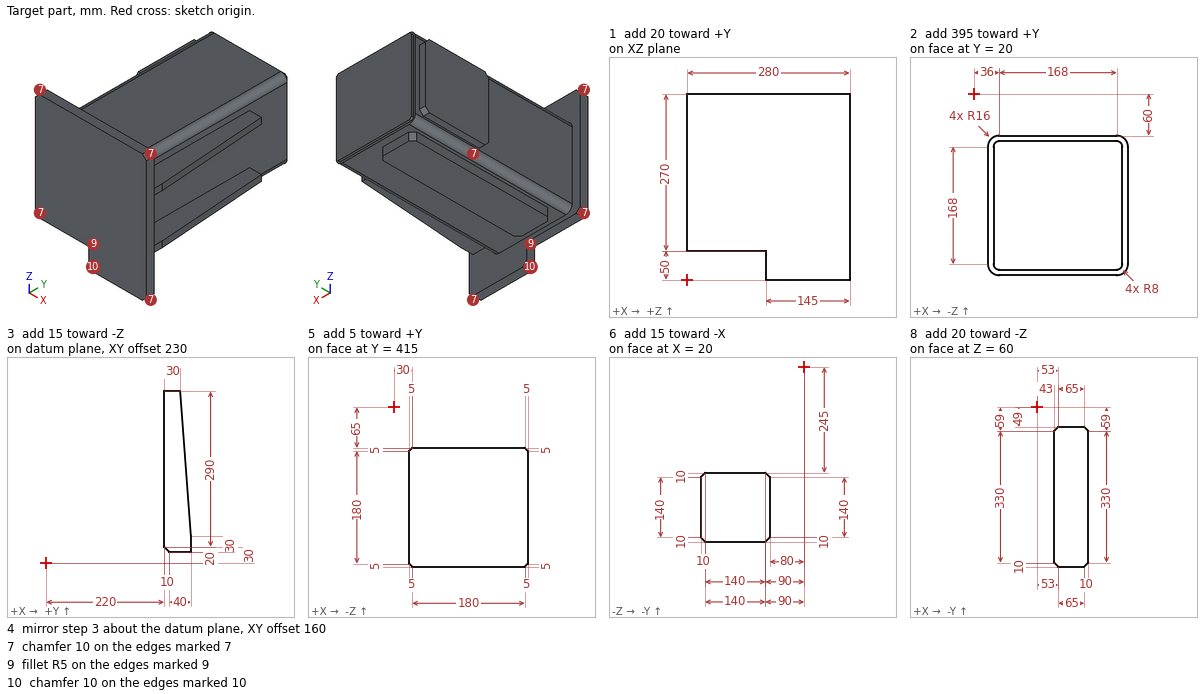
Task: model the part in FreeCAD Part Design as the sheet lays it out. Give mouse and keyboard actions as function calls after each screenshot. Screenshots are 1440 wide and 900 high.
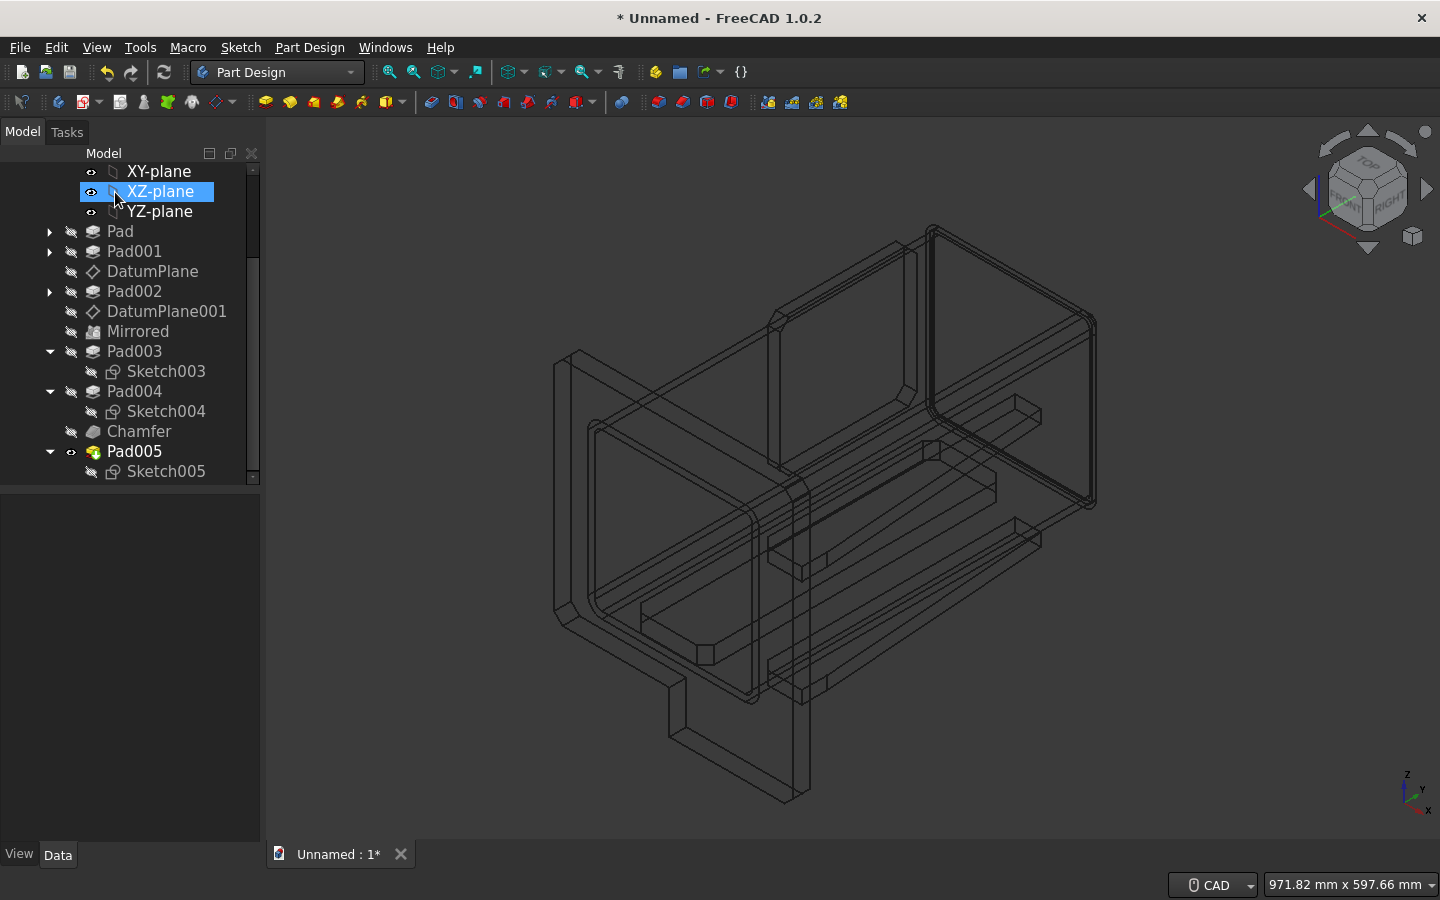
click(678, 682)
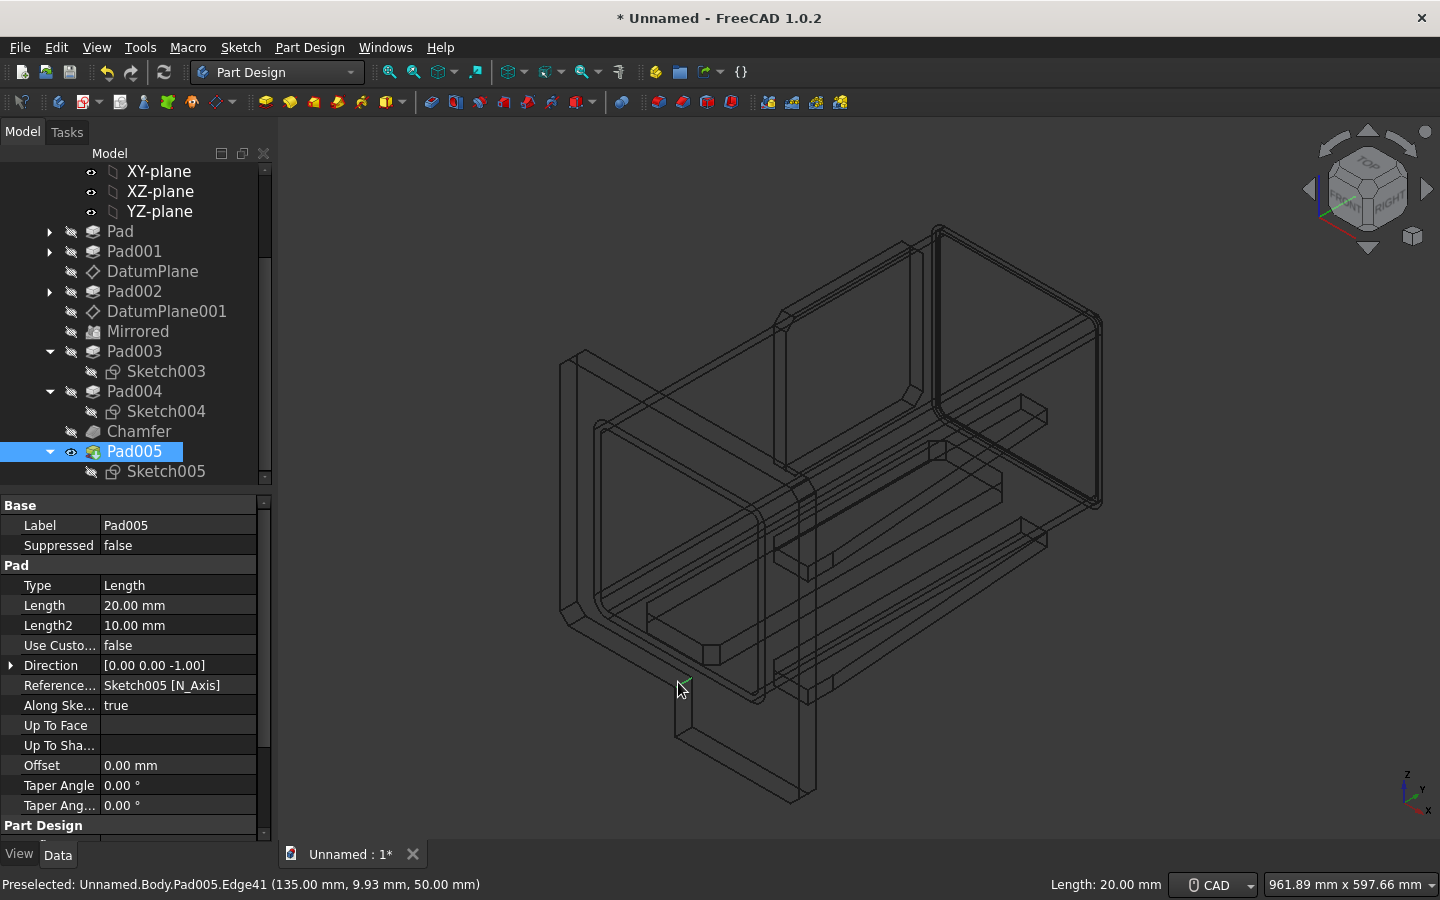
key(v)
key(1)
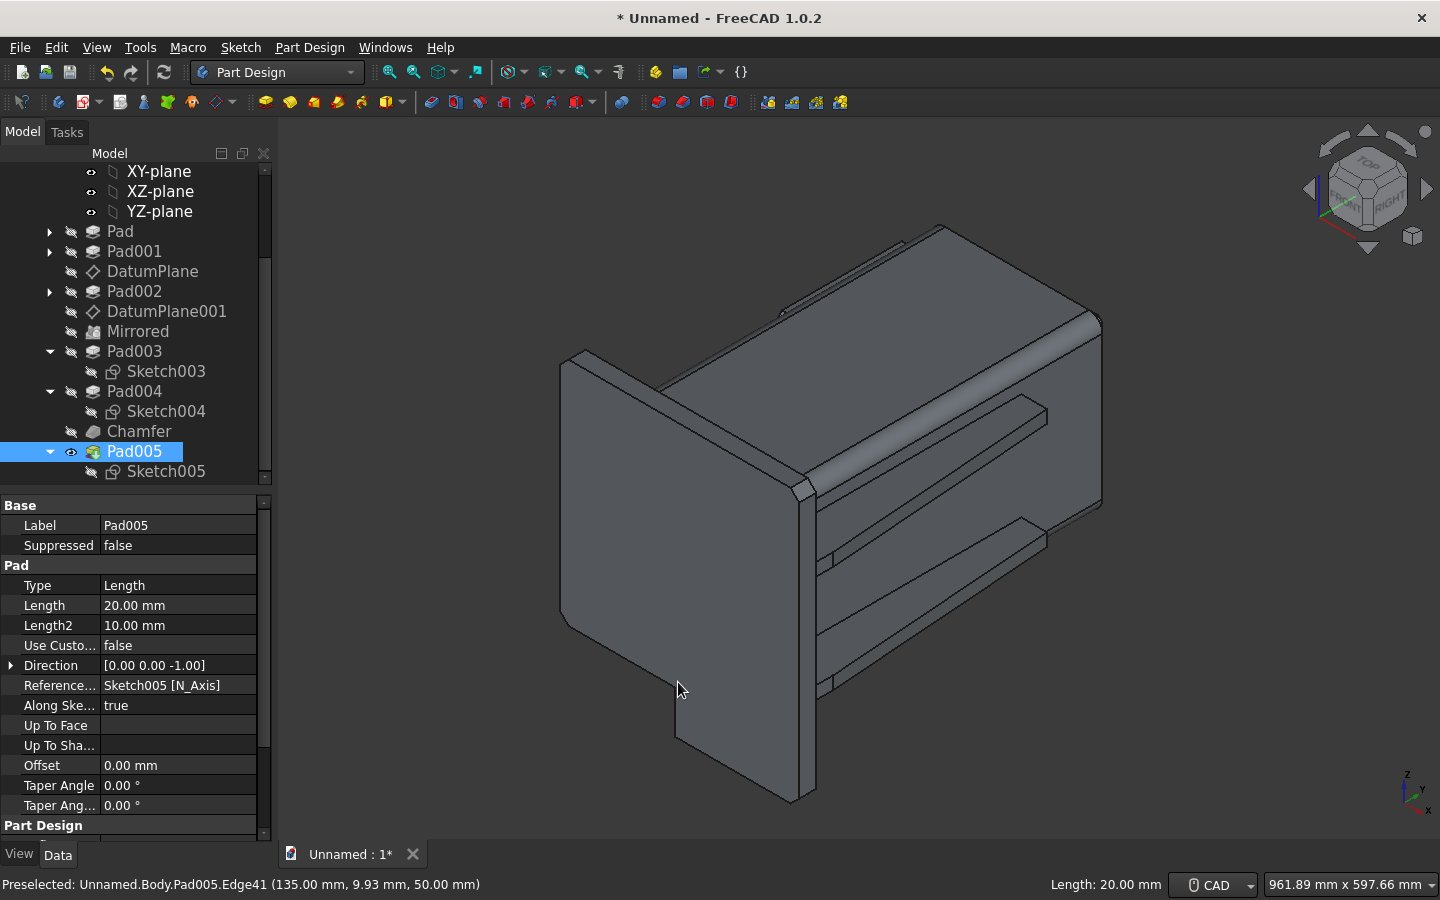
click(660, 102)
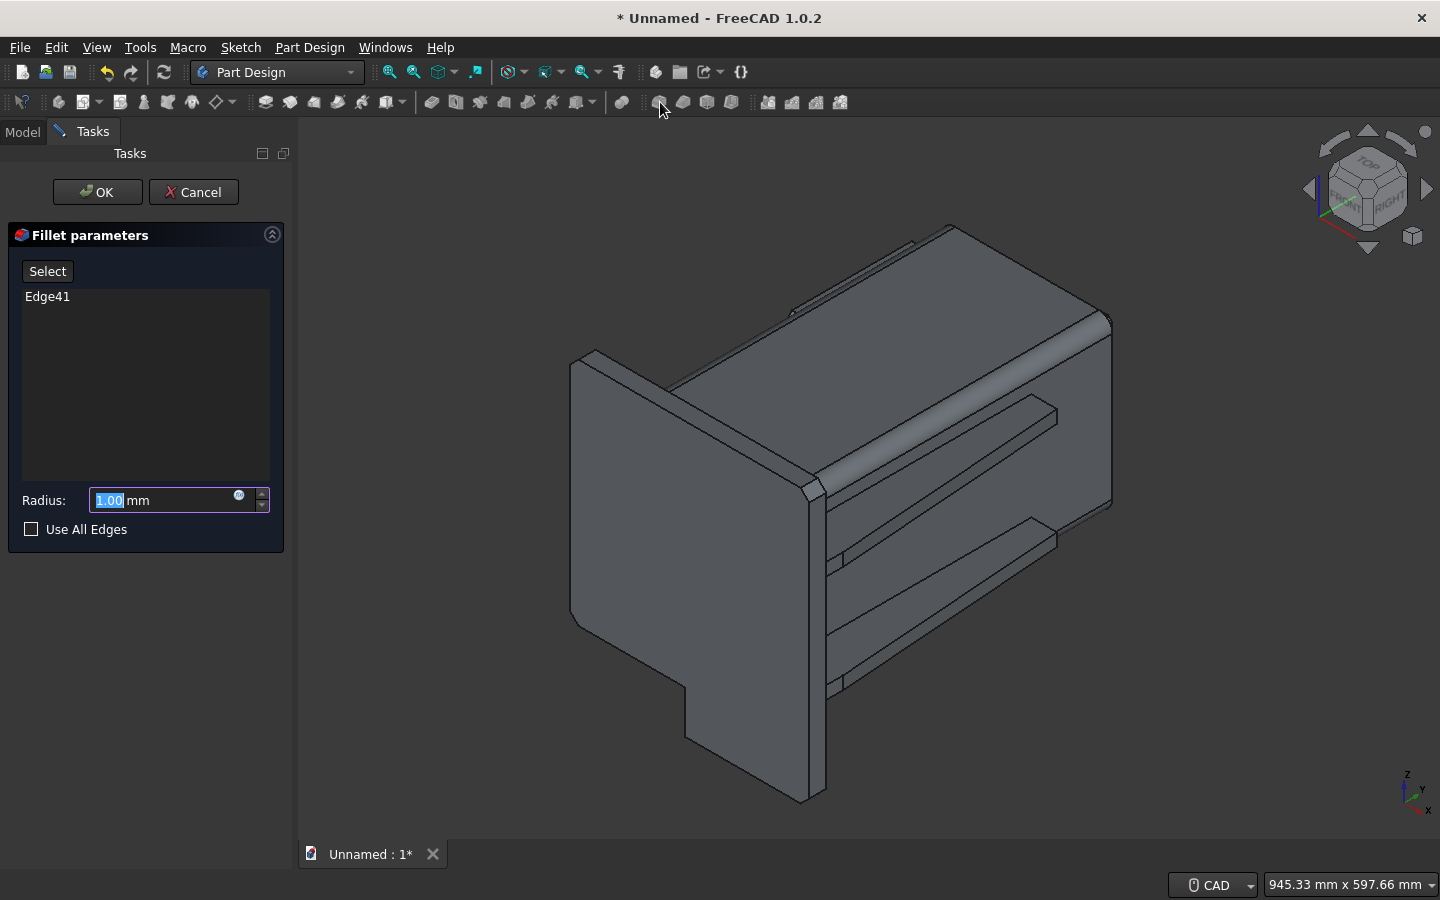
text(5)
key(Tab)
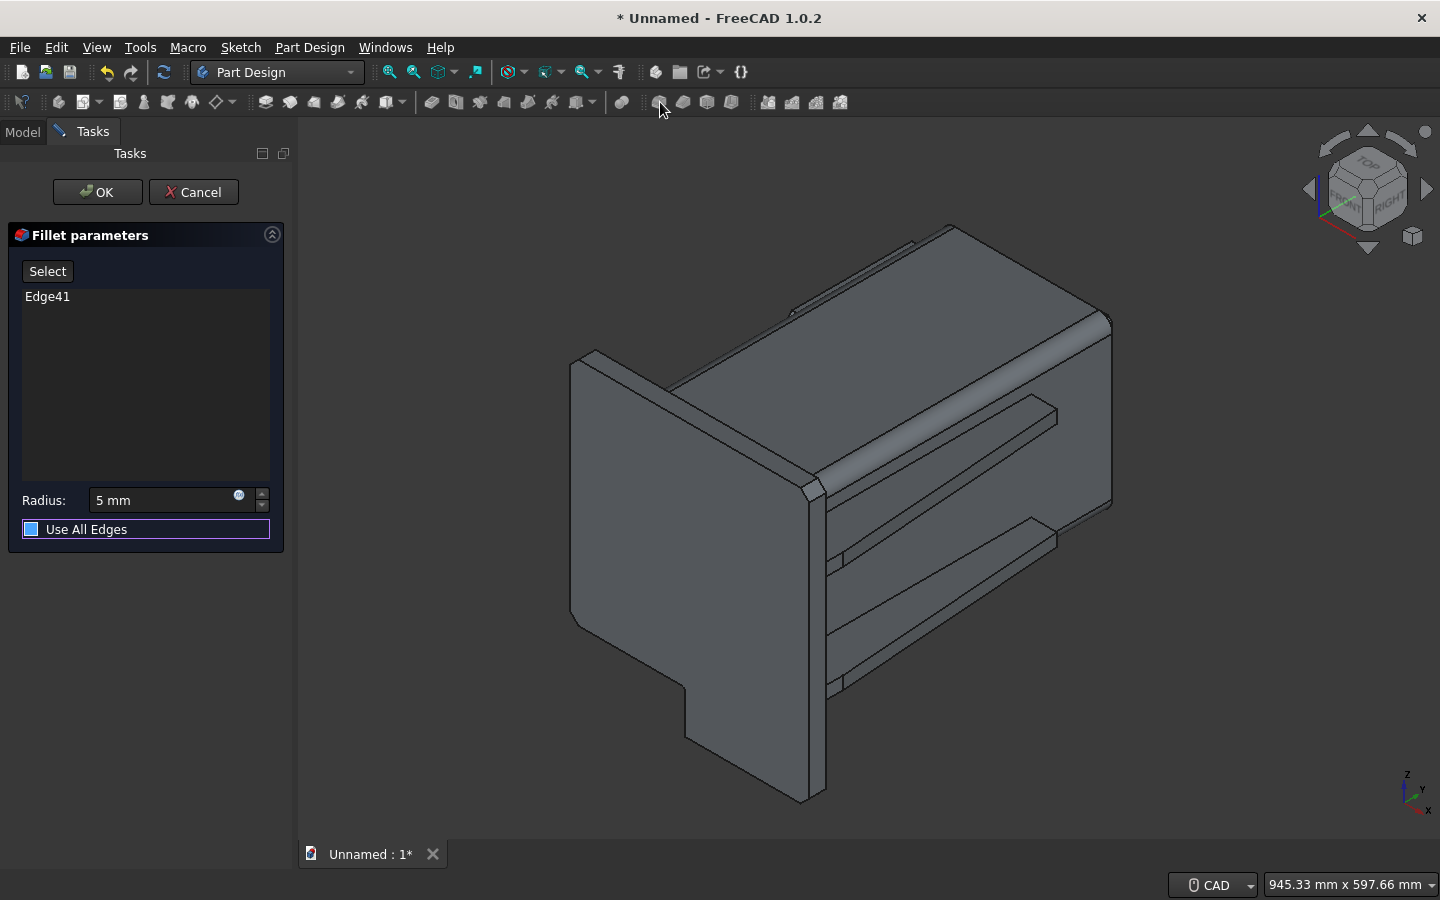
click(98, 192)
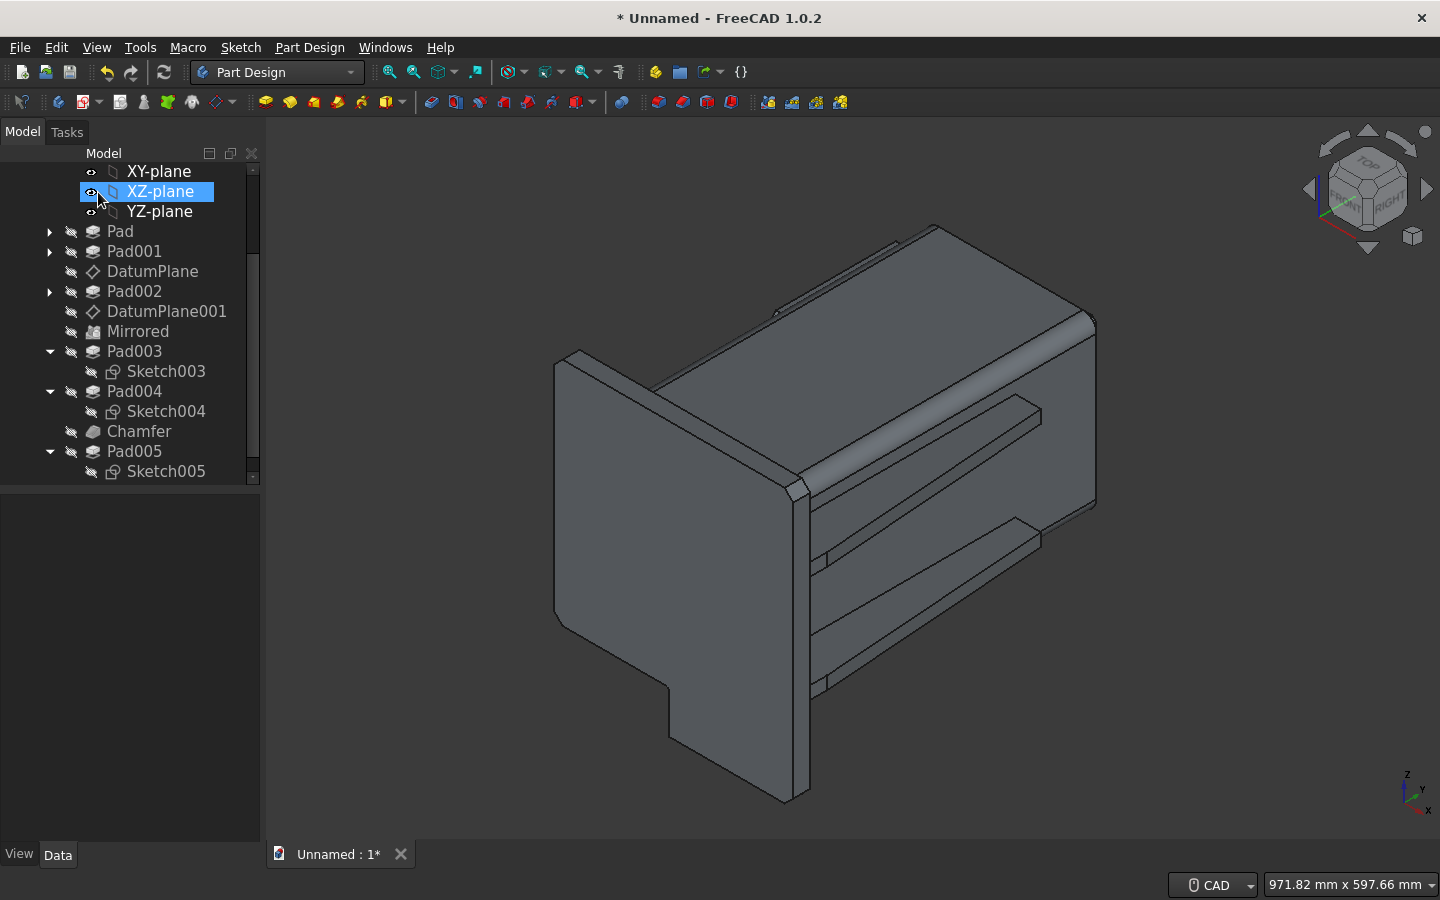
key(2)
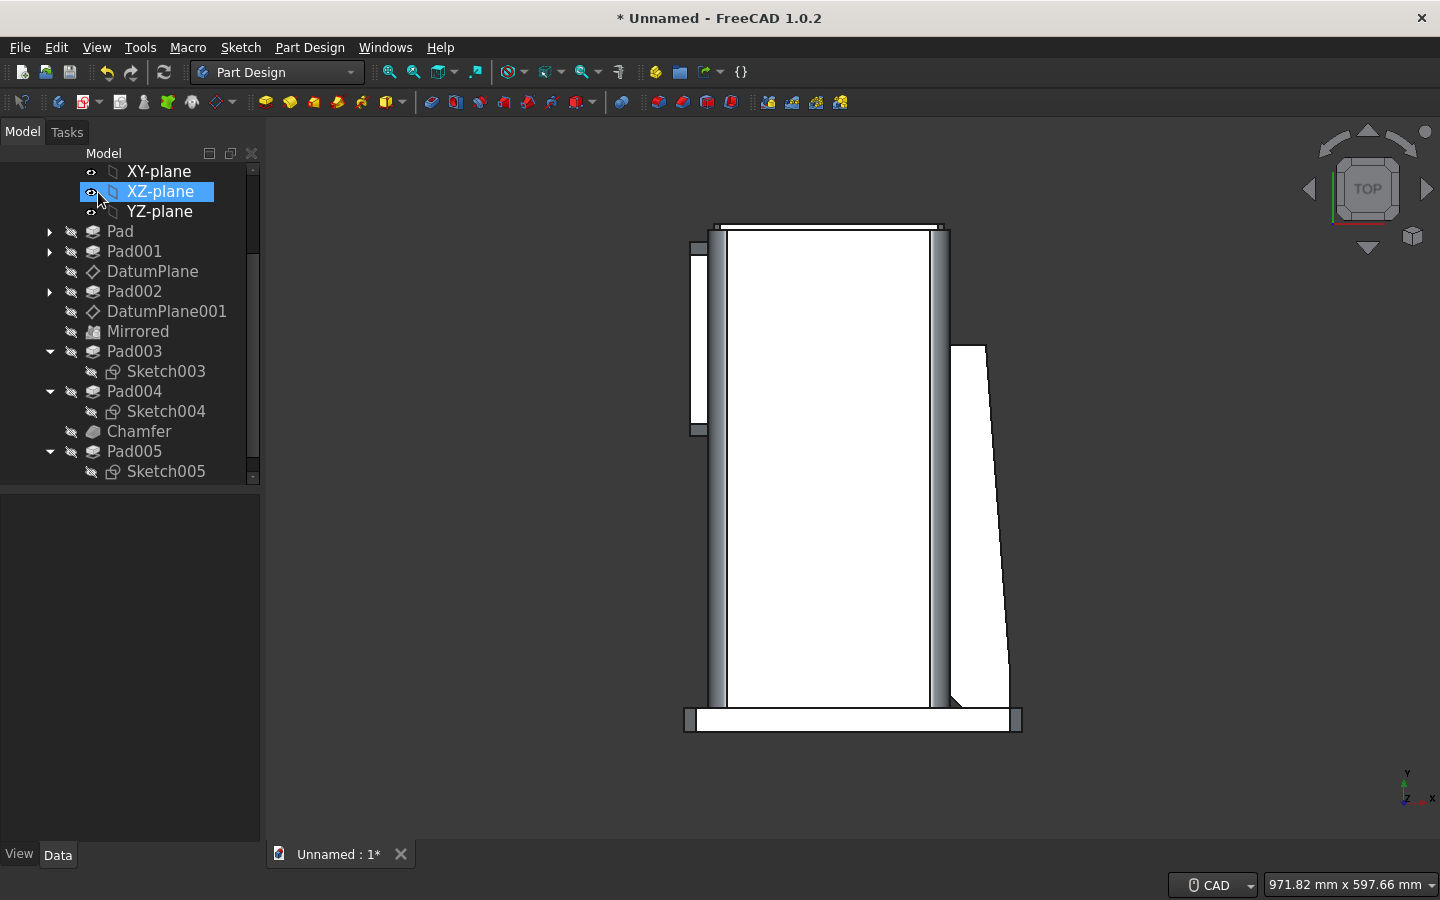
key(0)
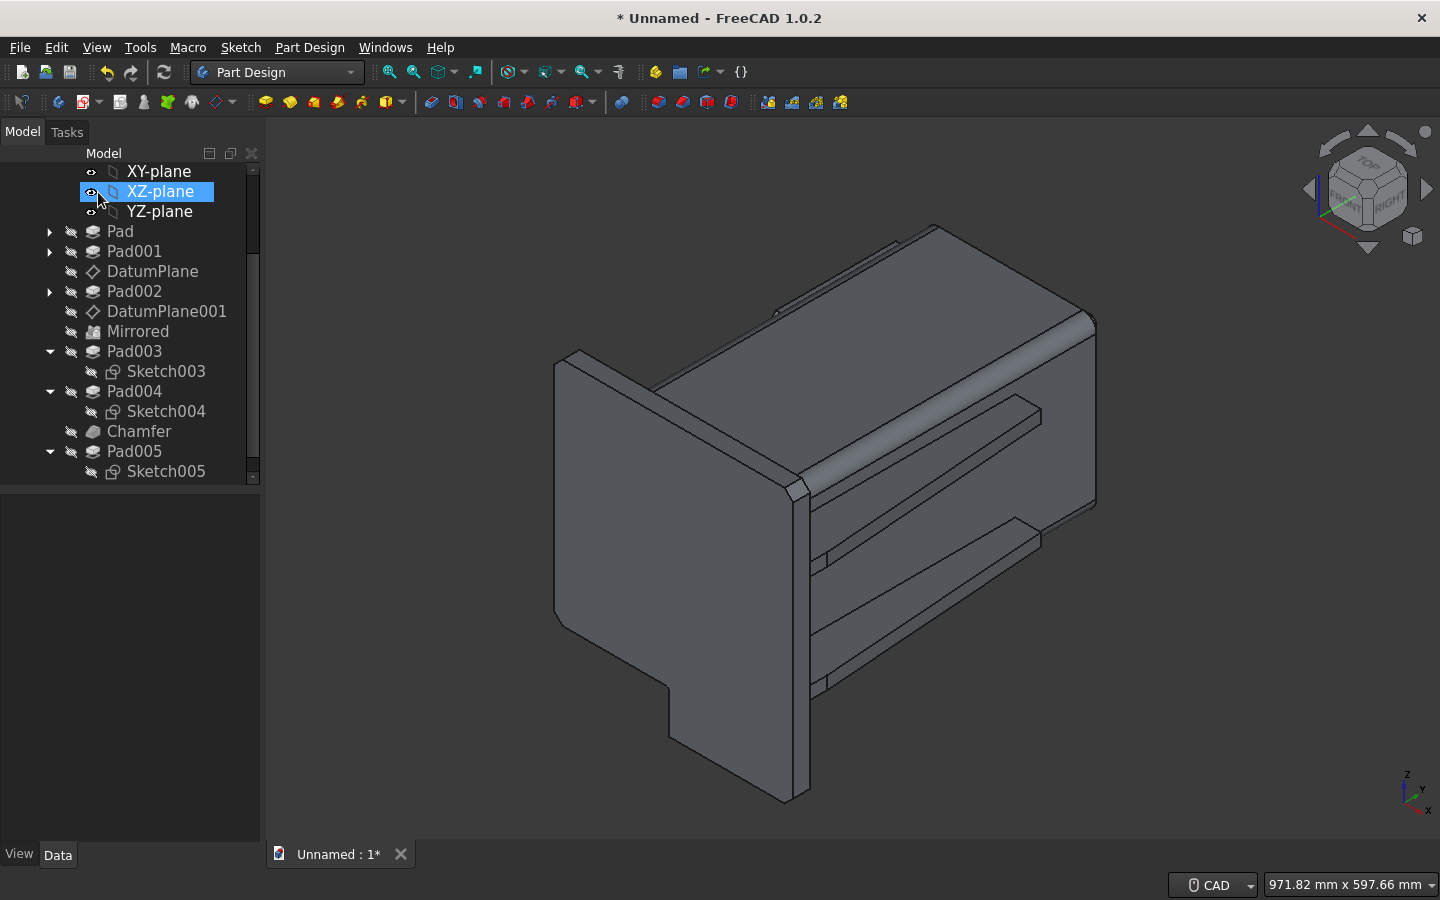
key(1)